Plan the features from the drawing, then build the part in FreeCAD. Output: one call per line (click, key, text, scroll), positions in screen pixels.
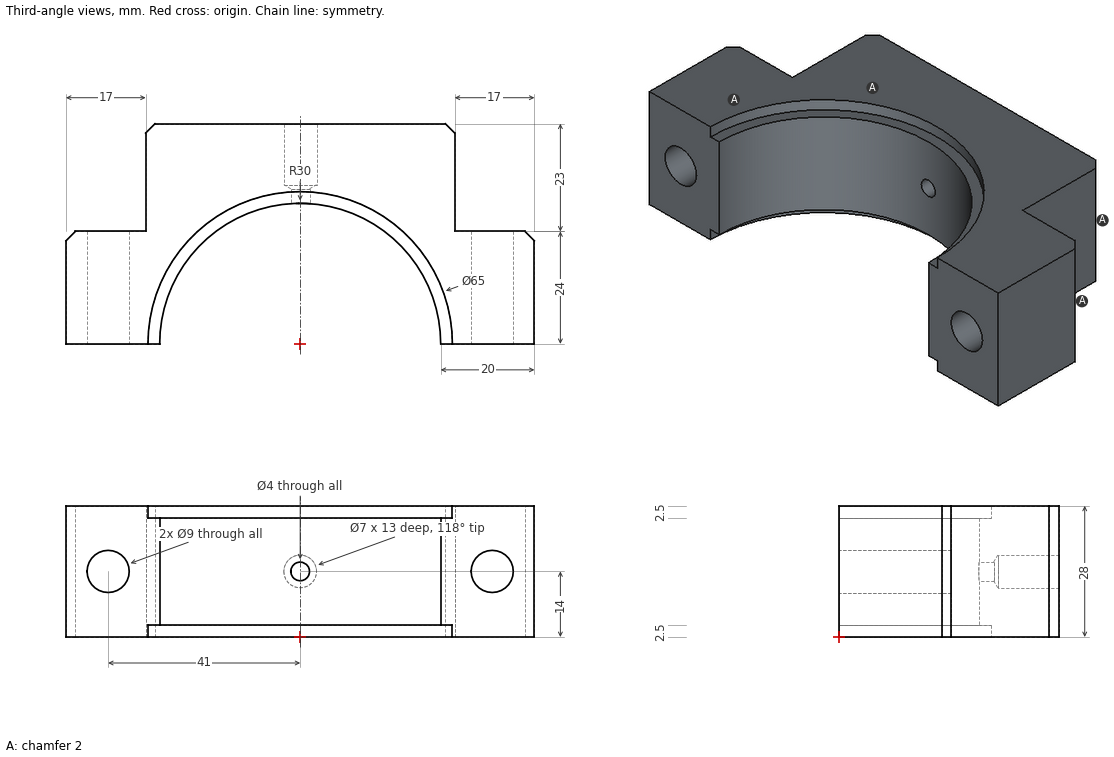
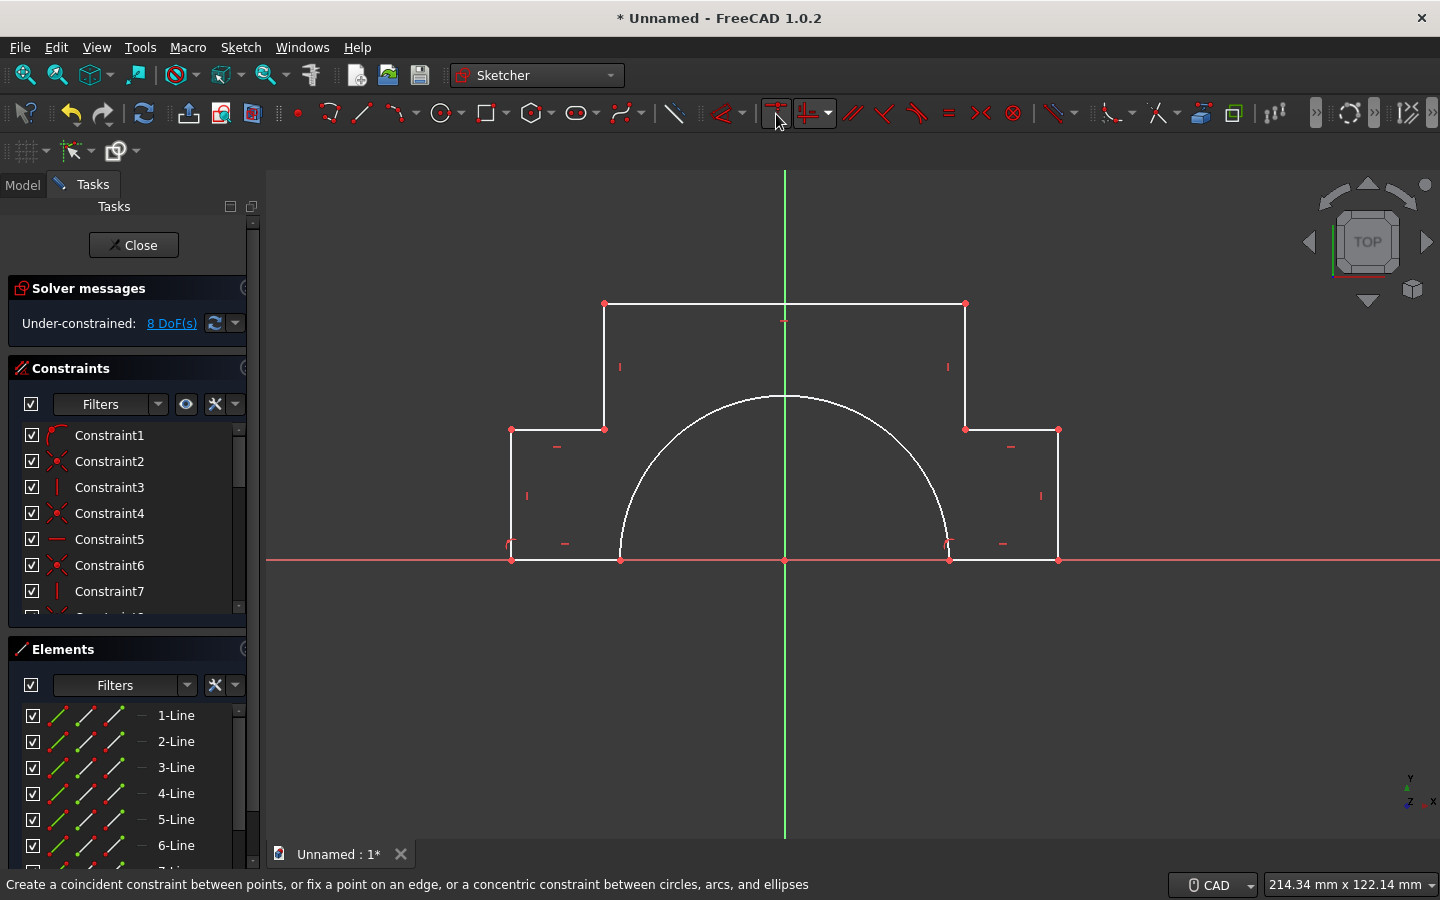
click(965, 430)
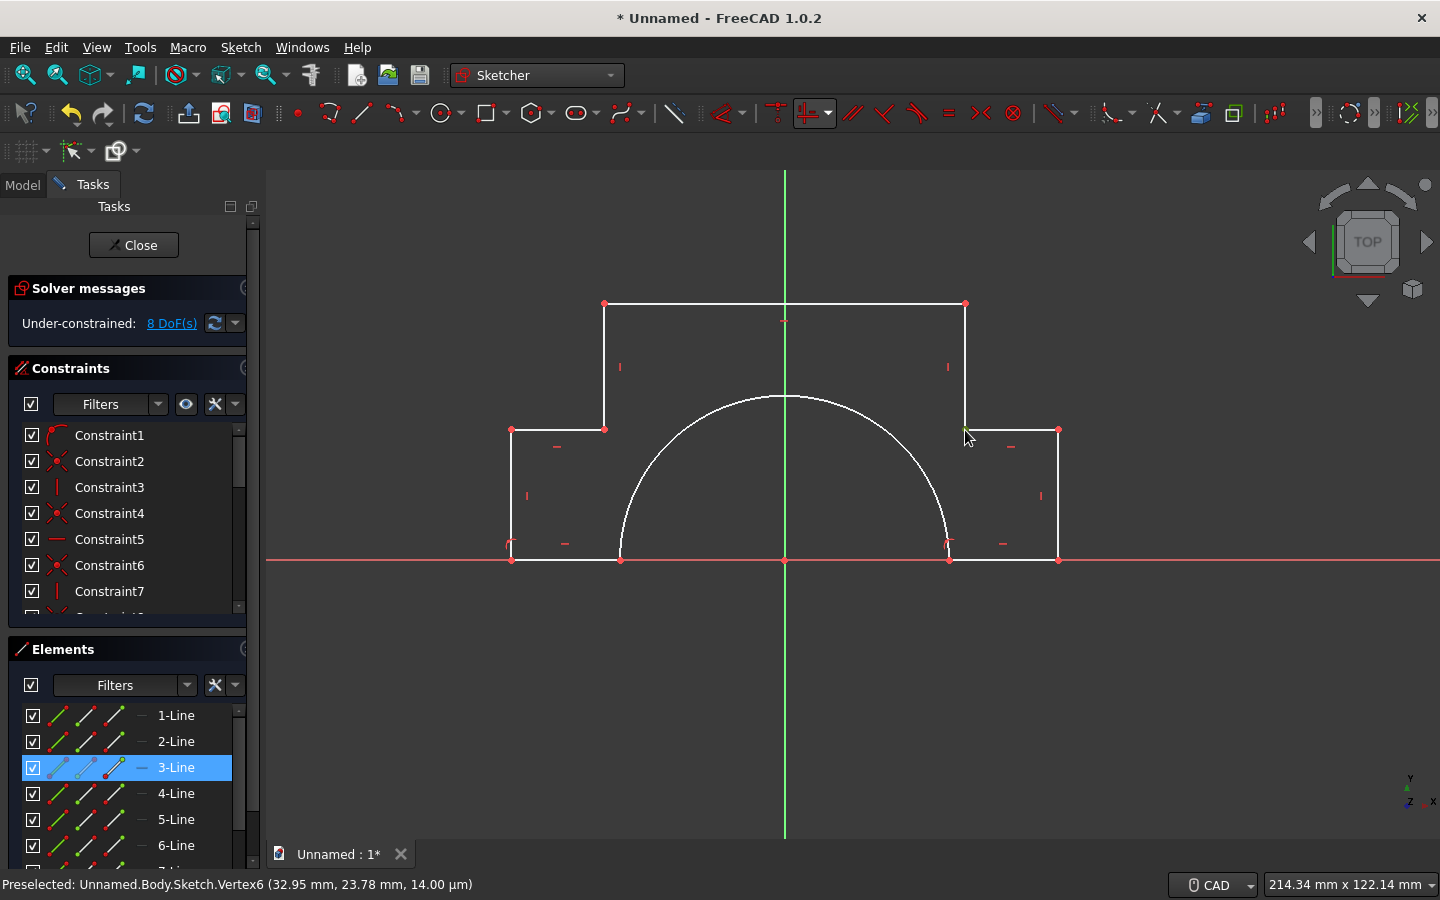
click(604, 430)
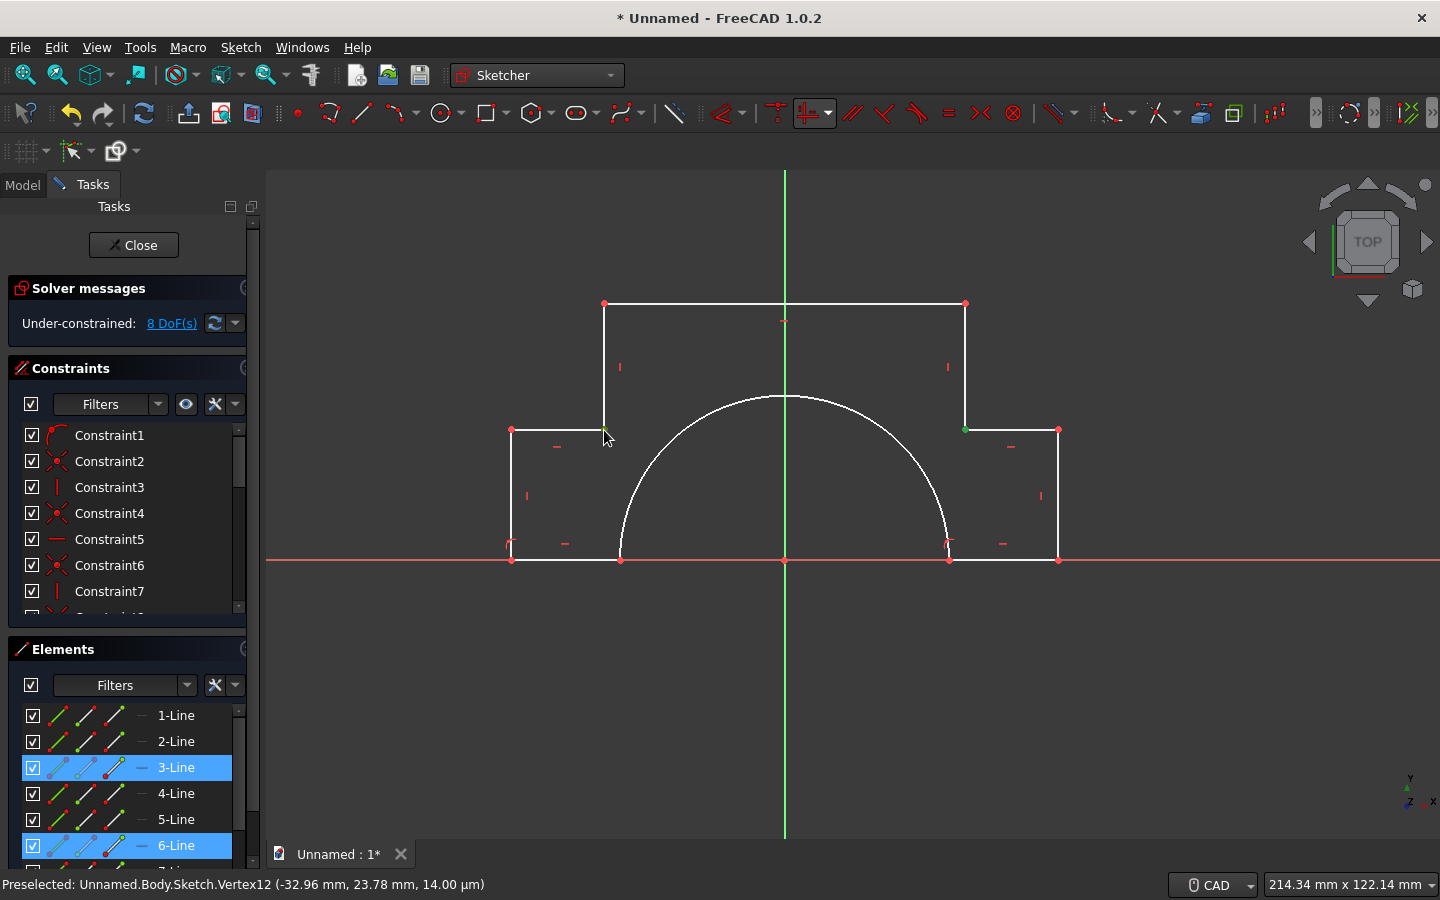
click(785, 767)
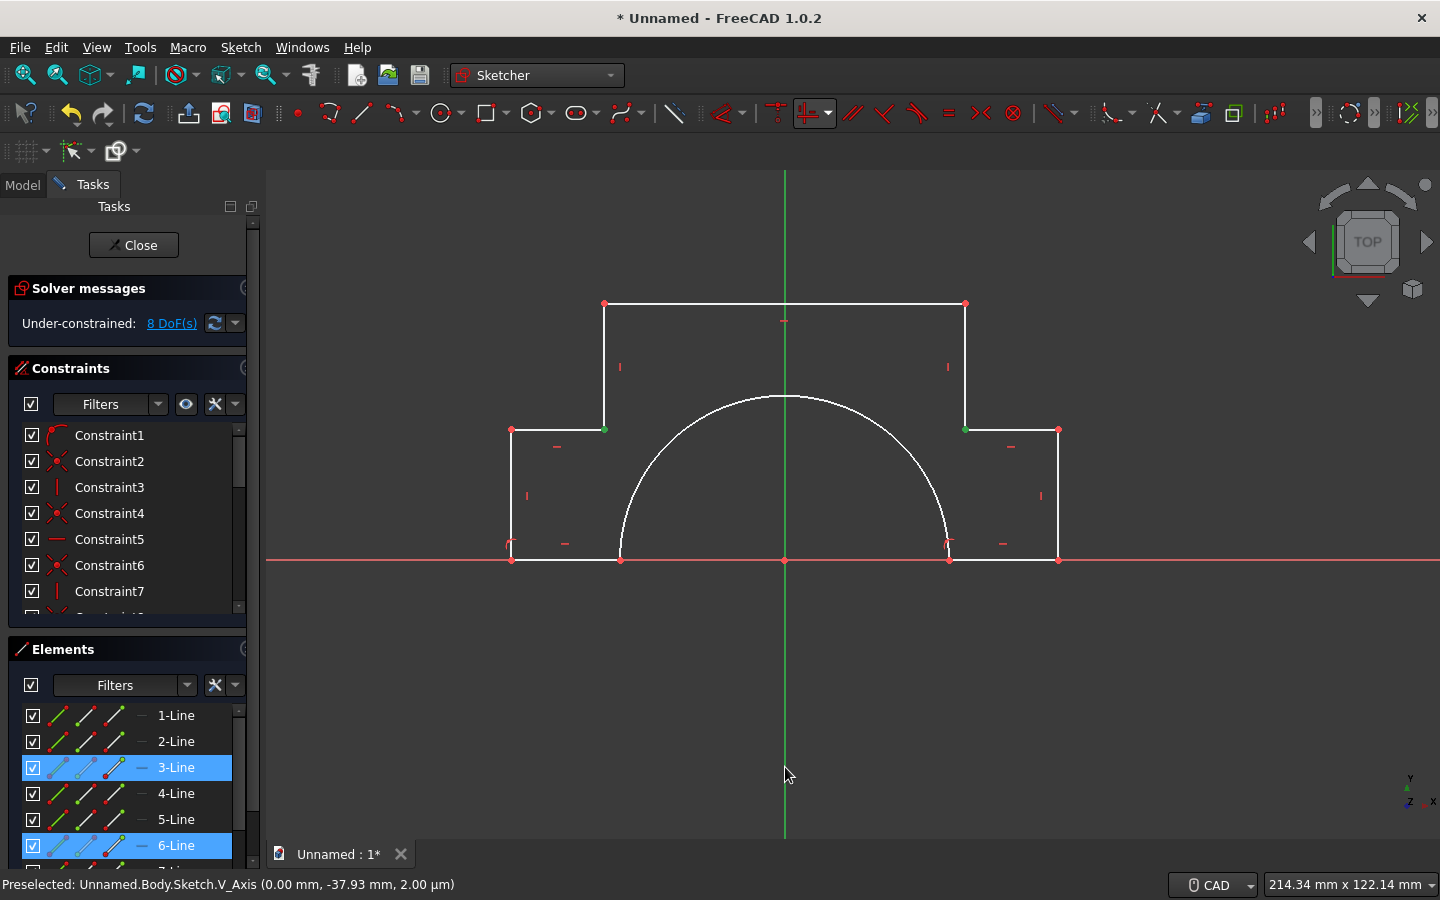
click(982, 114)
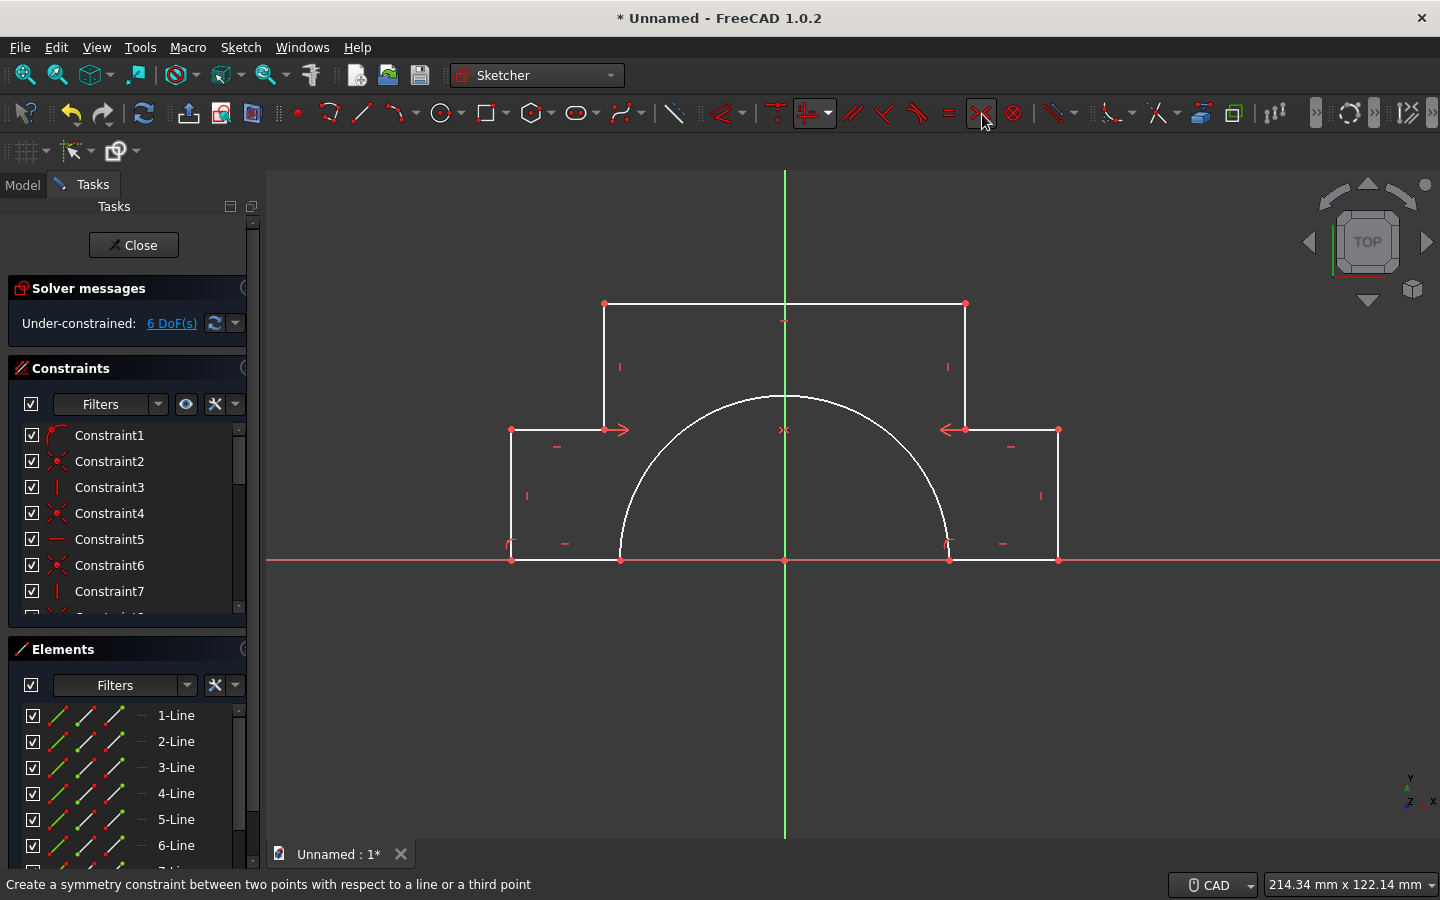
click(722, 114)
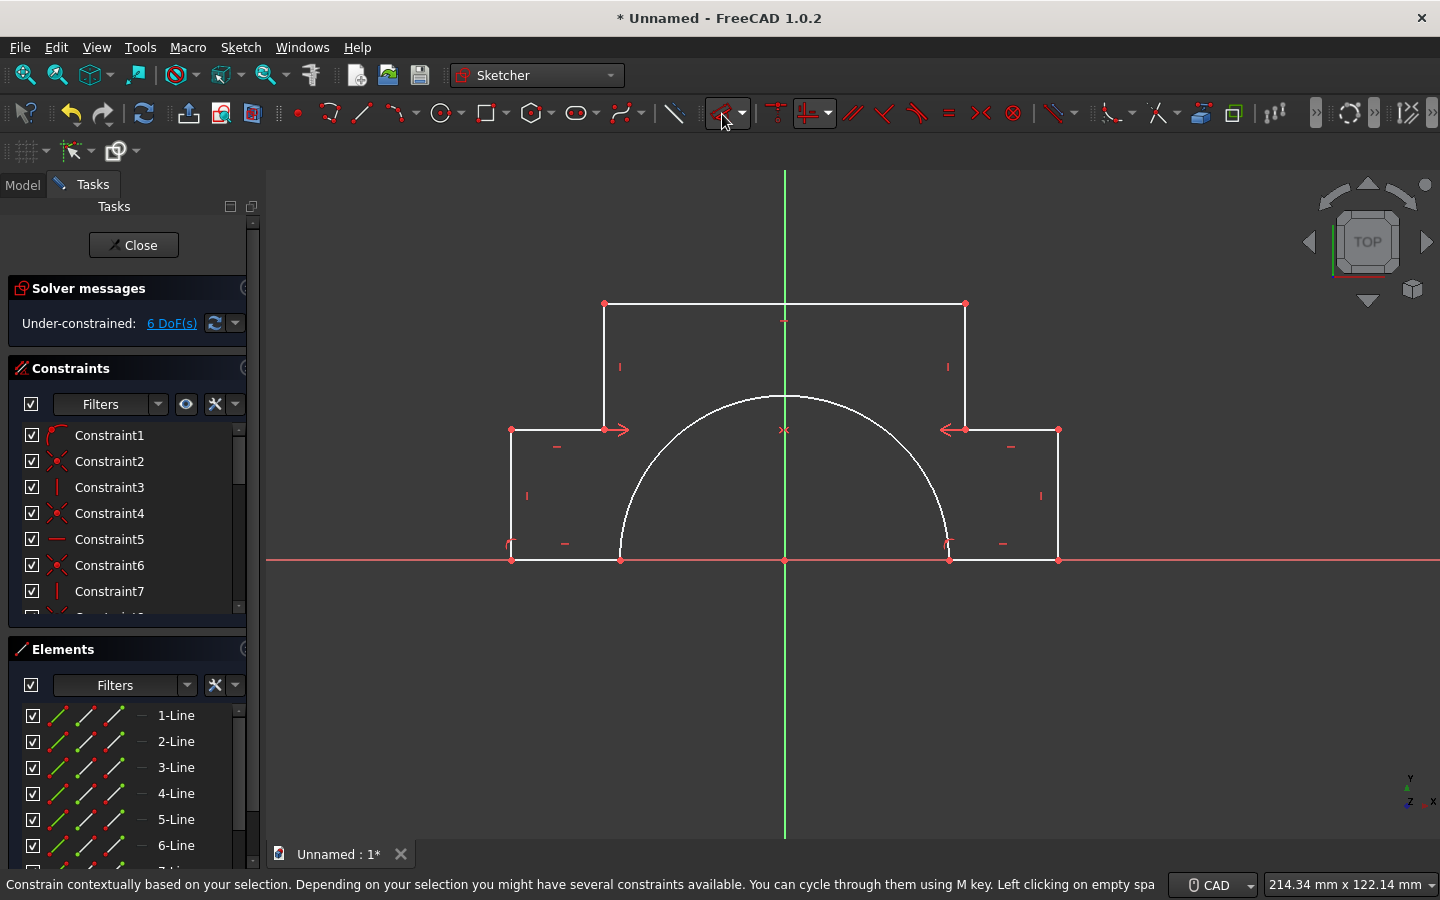
click(881, 427)
click(900, 401)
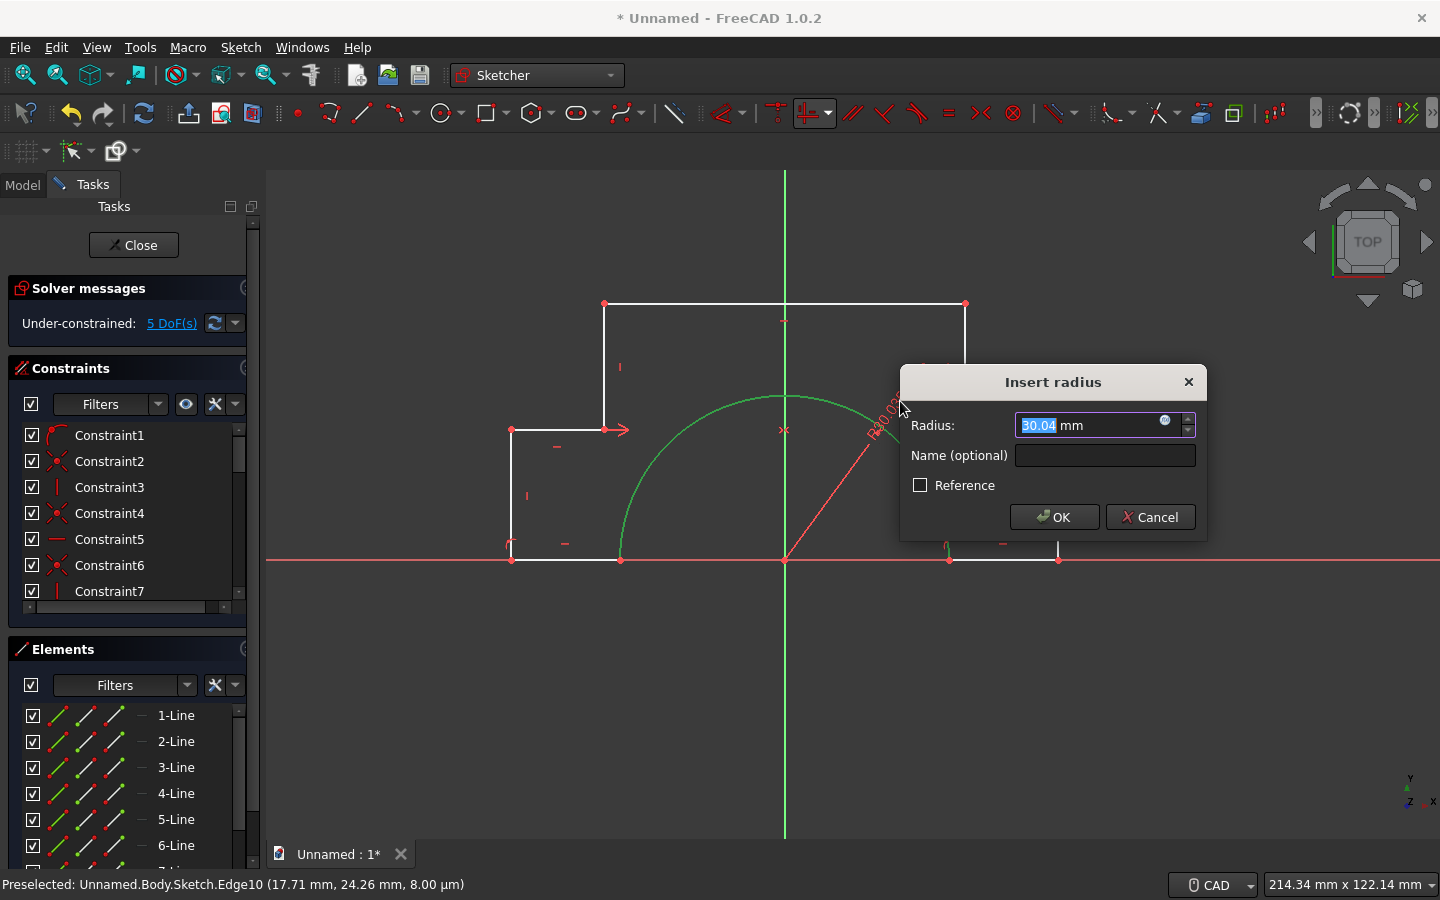
text(30)
key(Return)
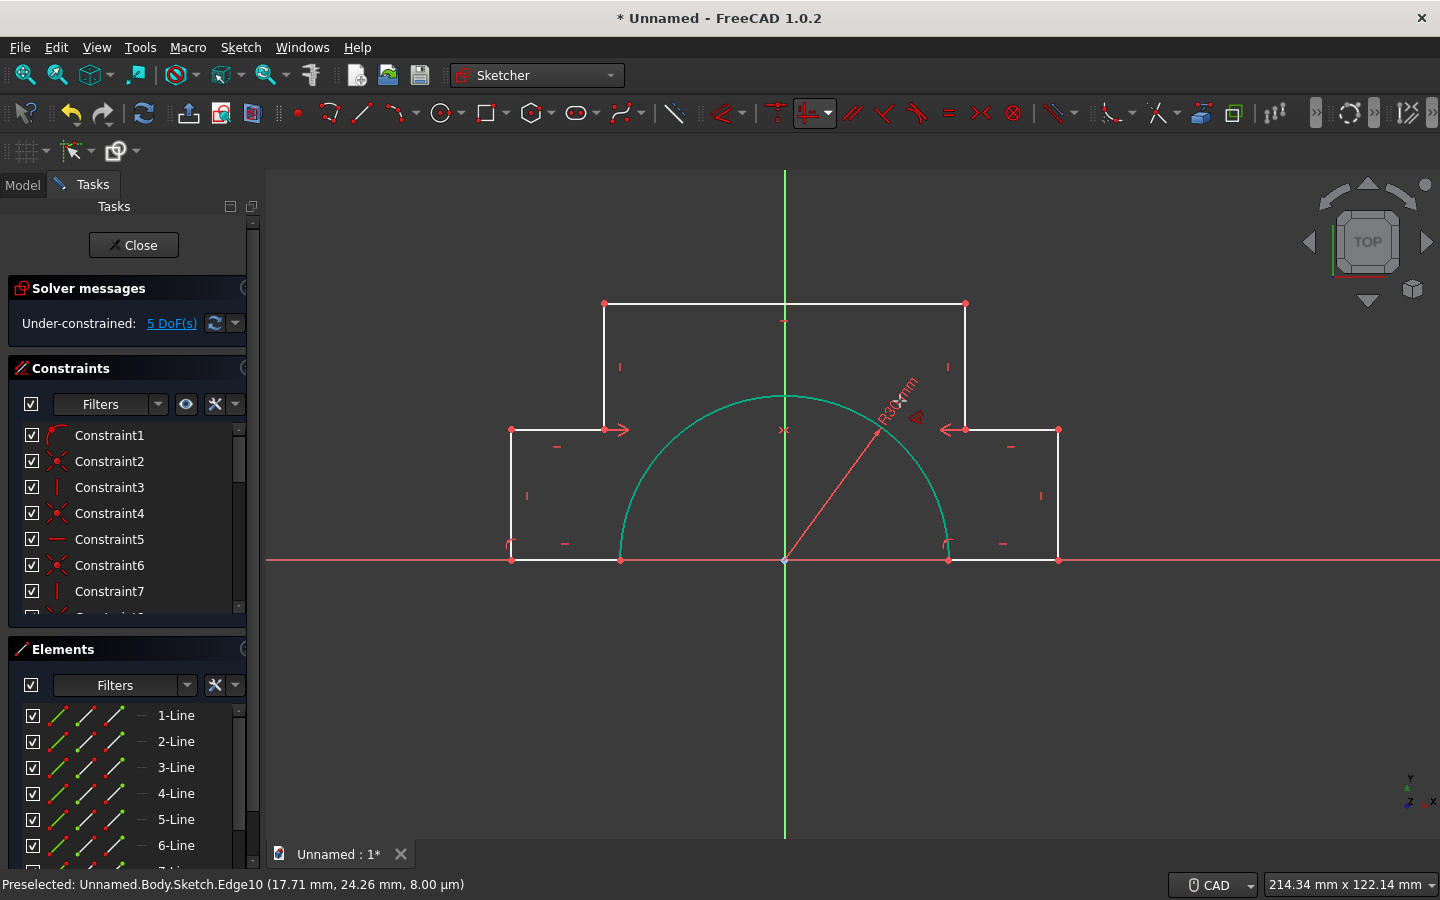
click(982, 560)
click(1003, 594)